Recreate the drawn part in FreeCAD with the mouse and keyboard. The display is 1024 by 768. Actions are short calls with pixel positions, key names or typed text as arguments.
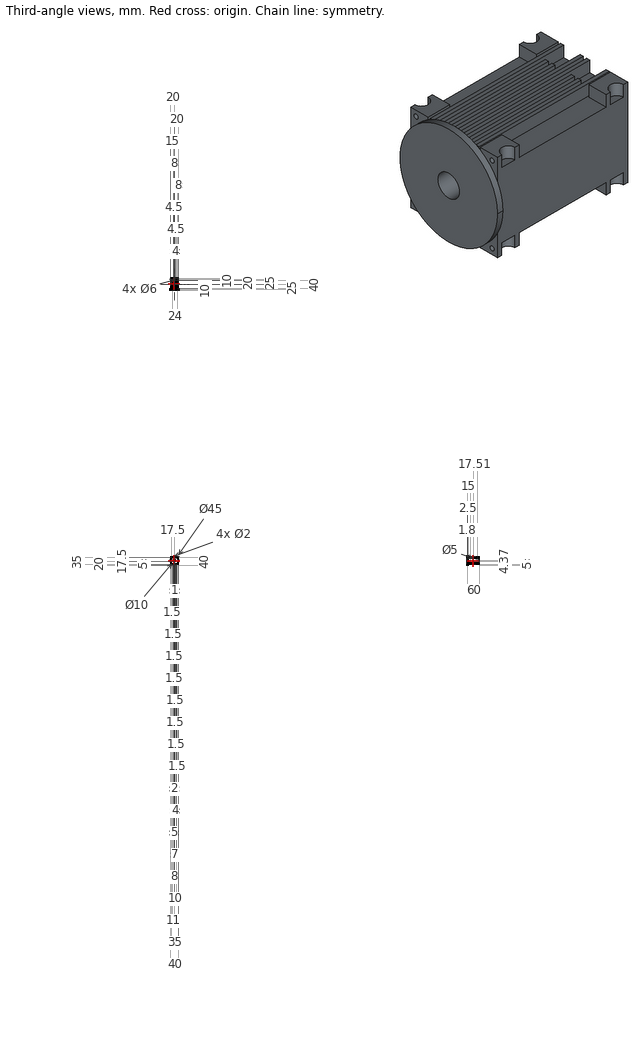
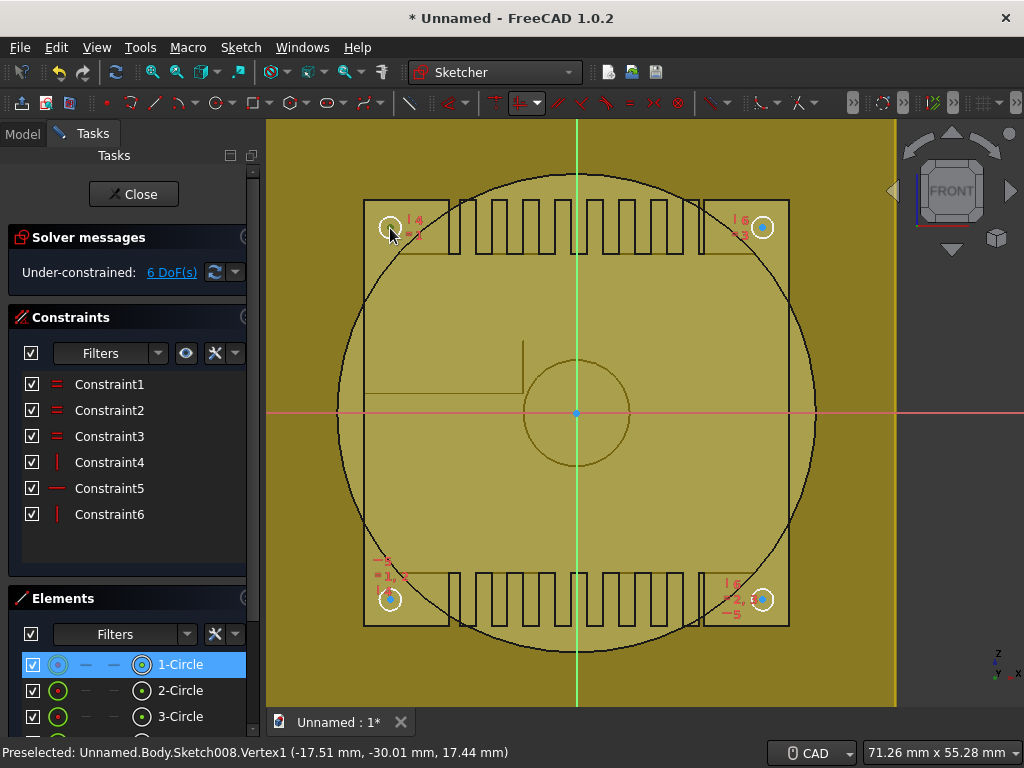
click(763, 228)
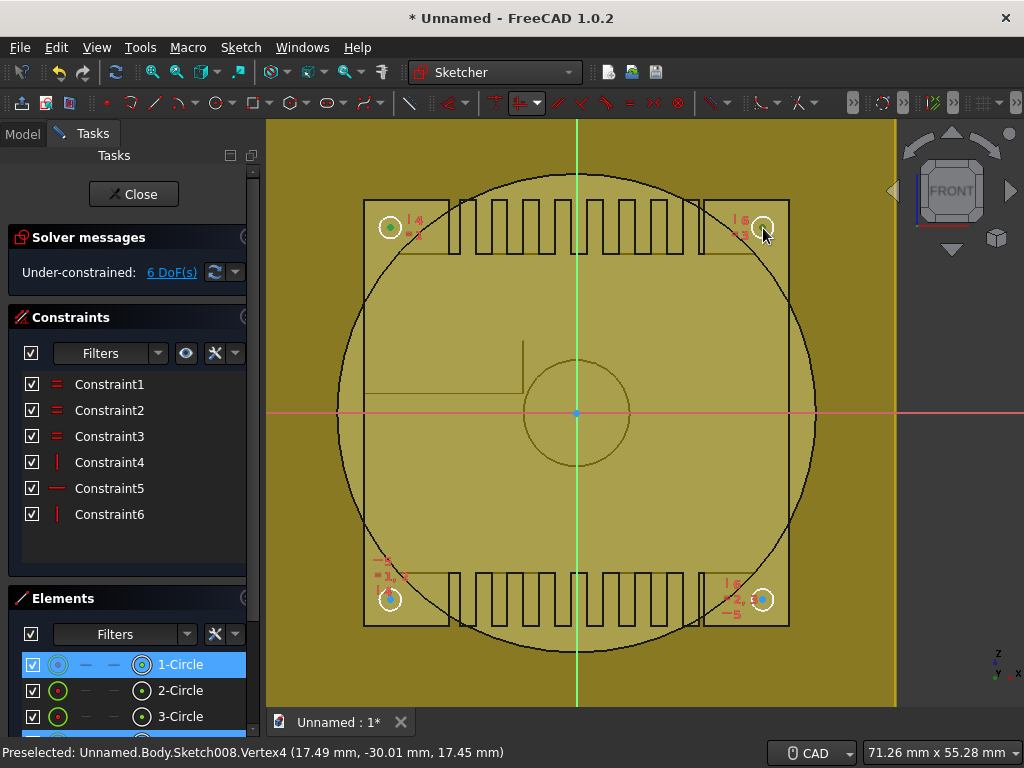
key(h)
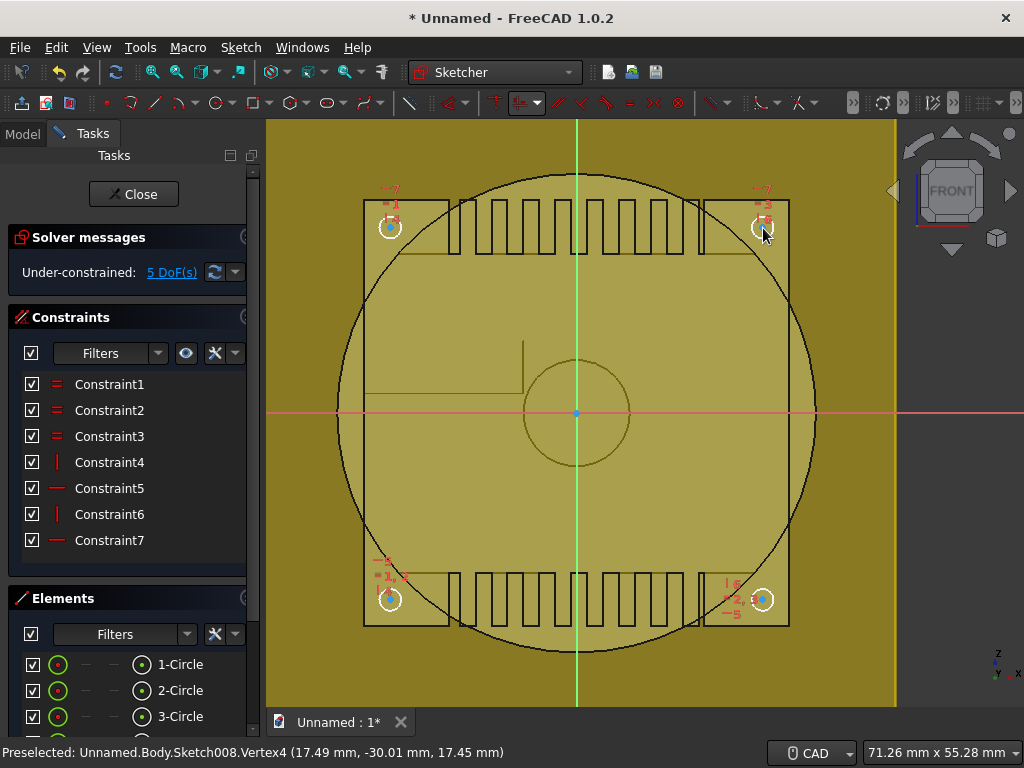
key(d)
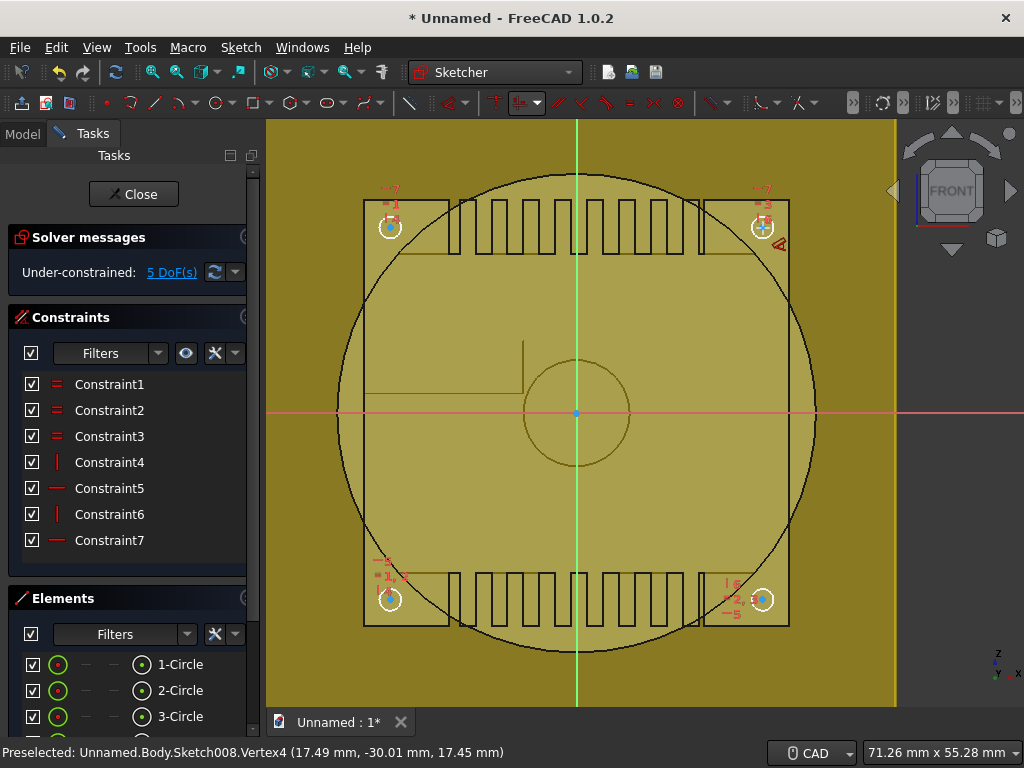
scroll(398, 220, up, 4)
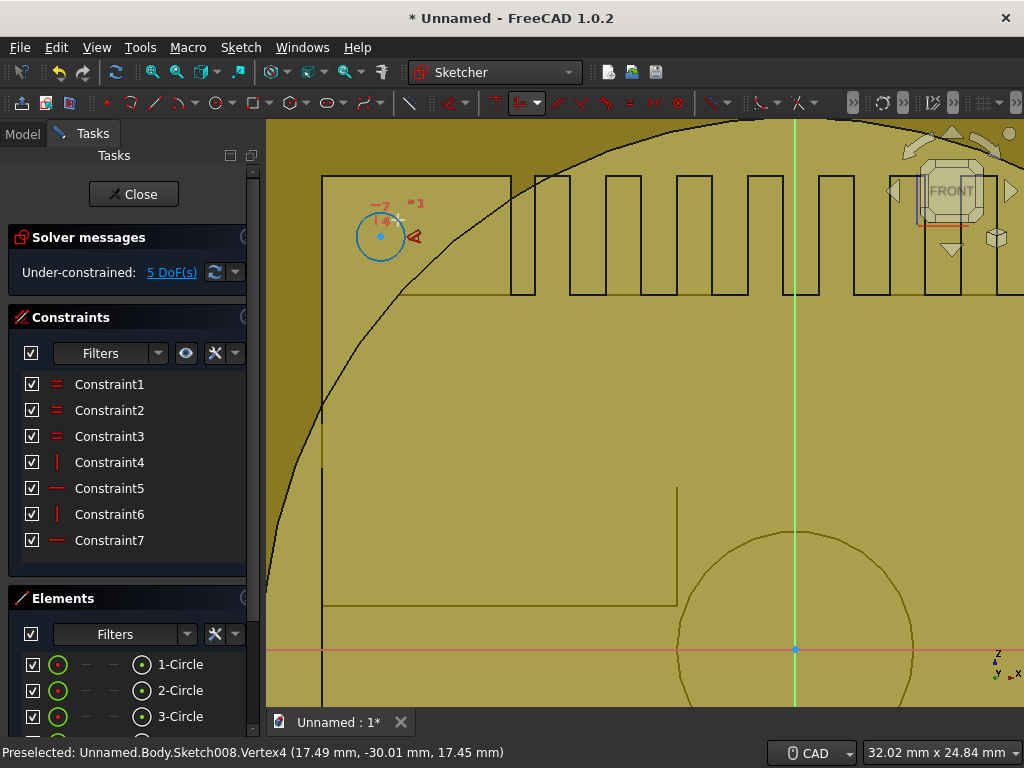
click(398, 220)
click(421, 198)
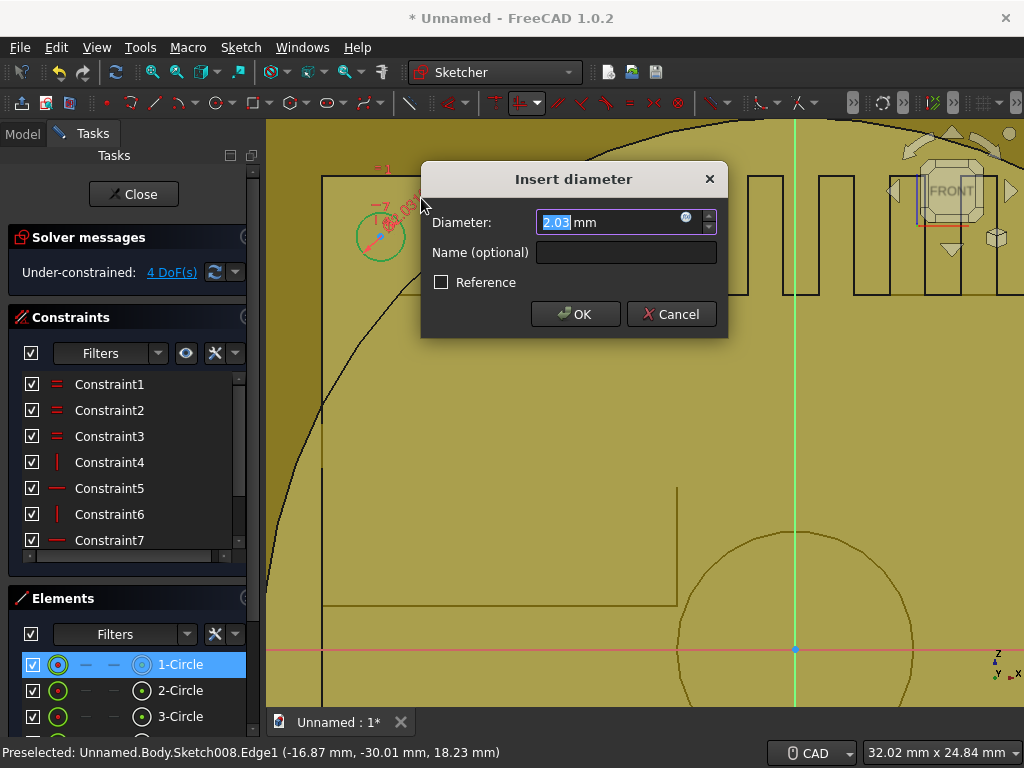
text(2)
key(Return)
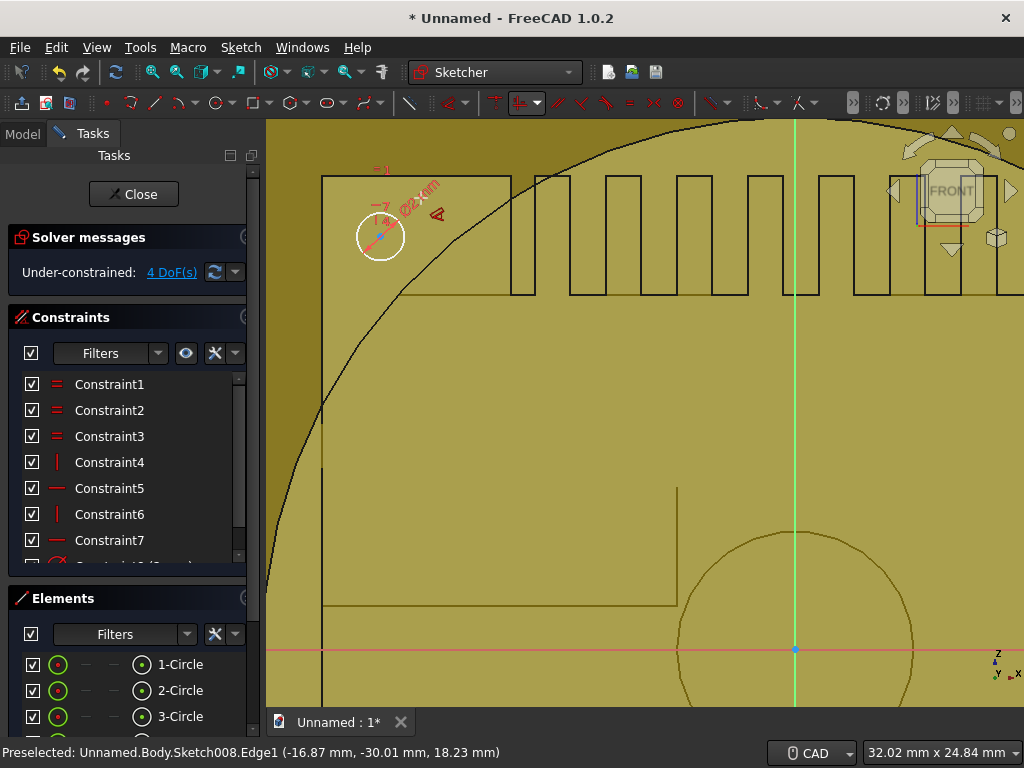
click(381, 237)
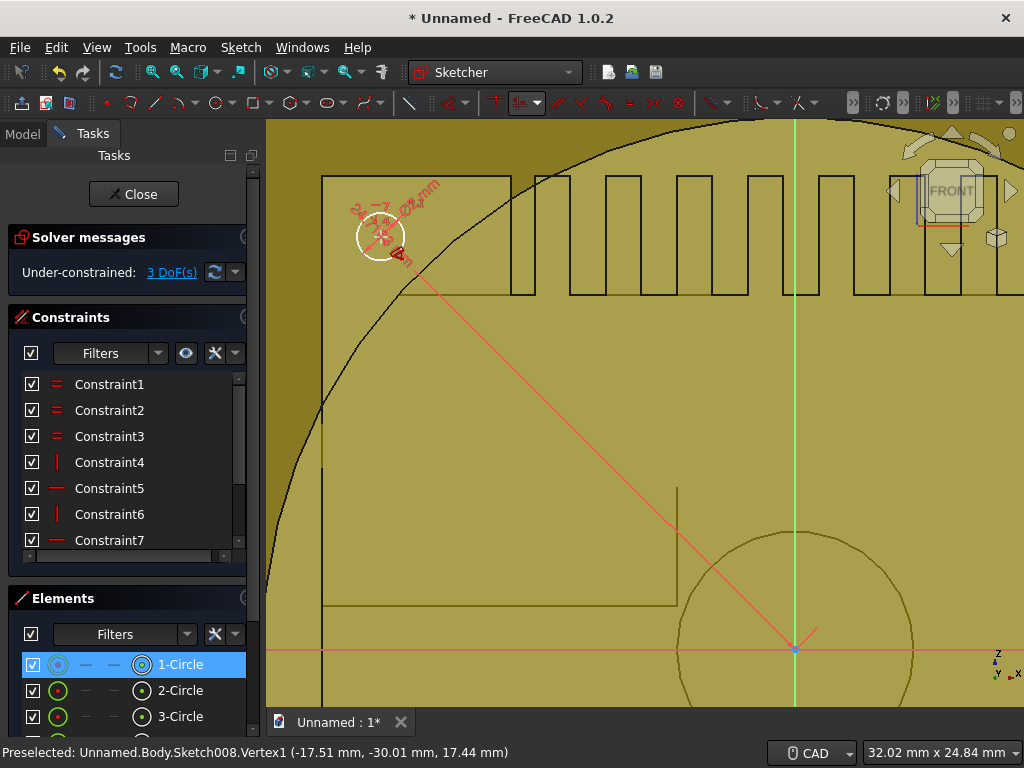
scroll(398, 220, down, 4)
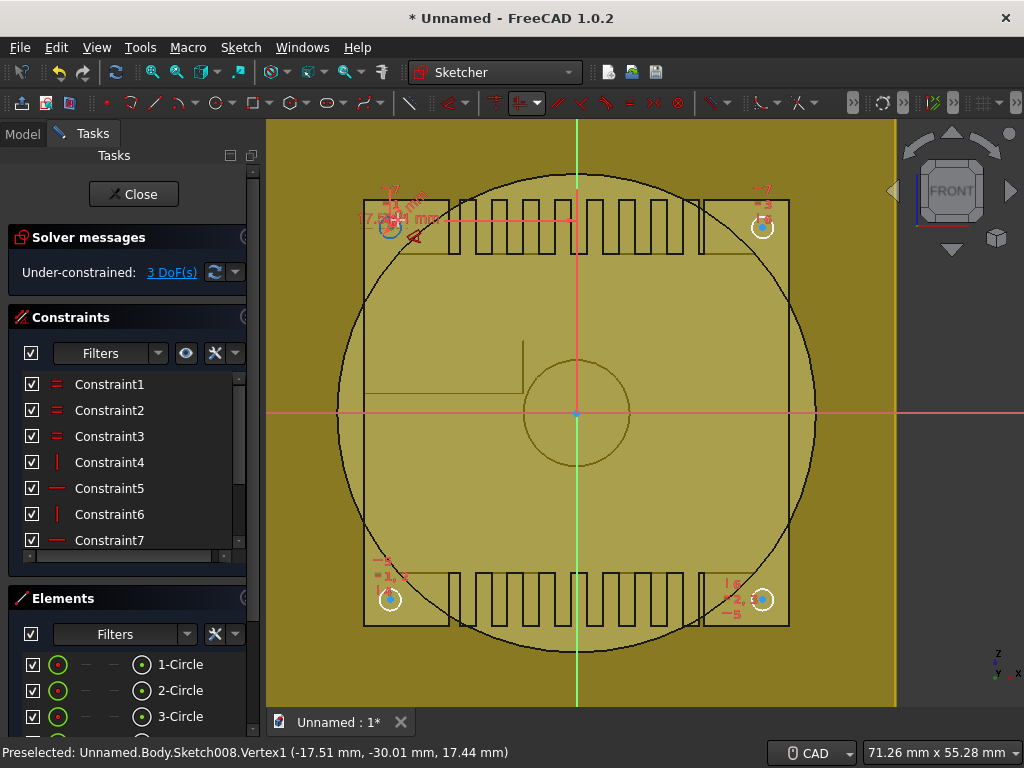
click(390, 600)
click(356, 328)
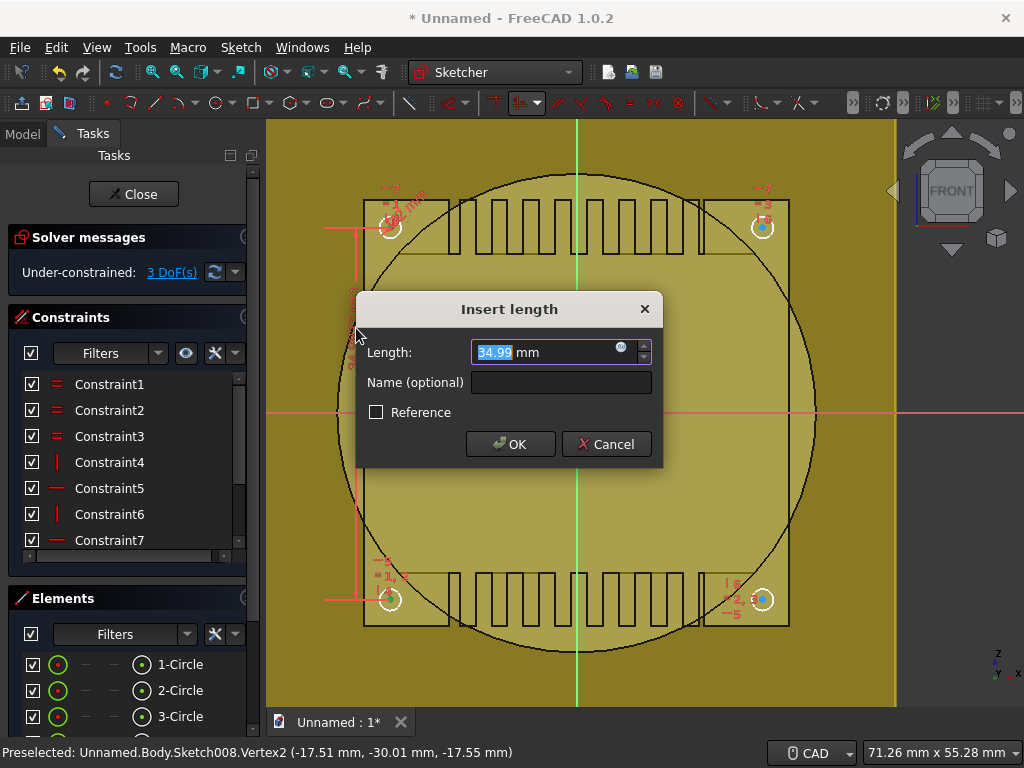
text(35)
key(Return)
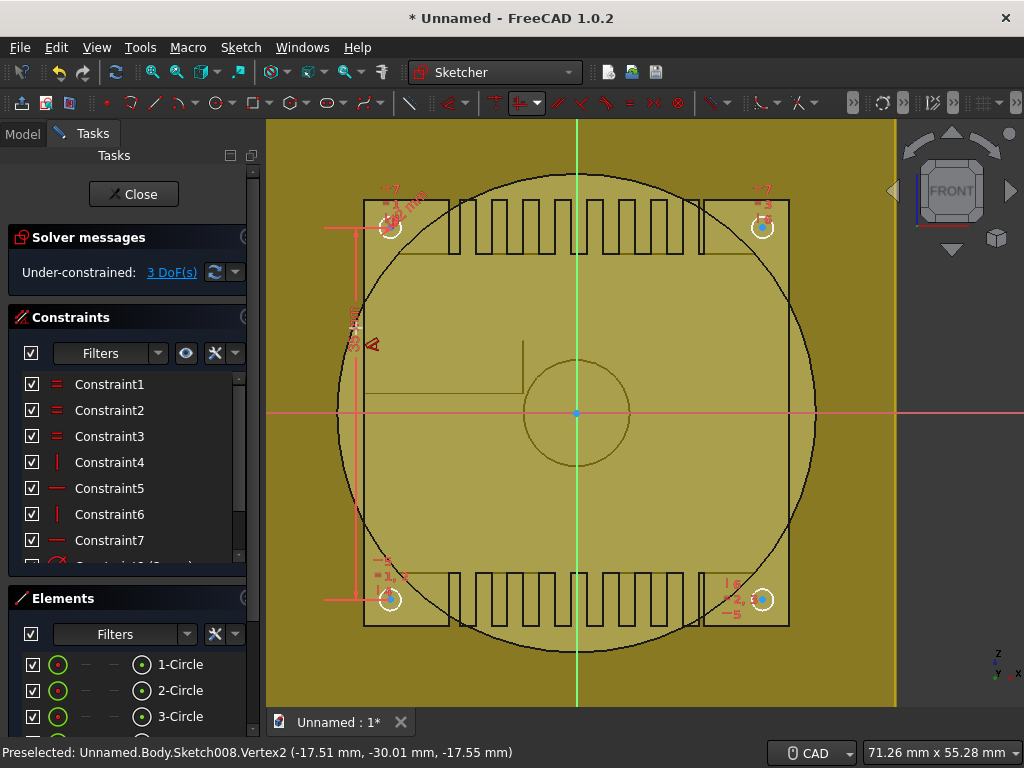
click(390, 600)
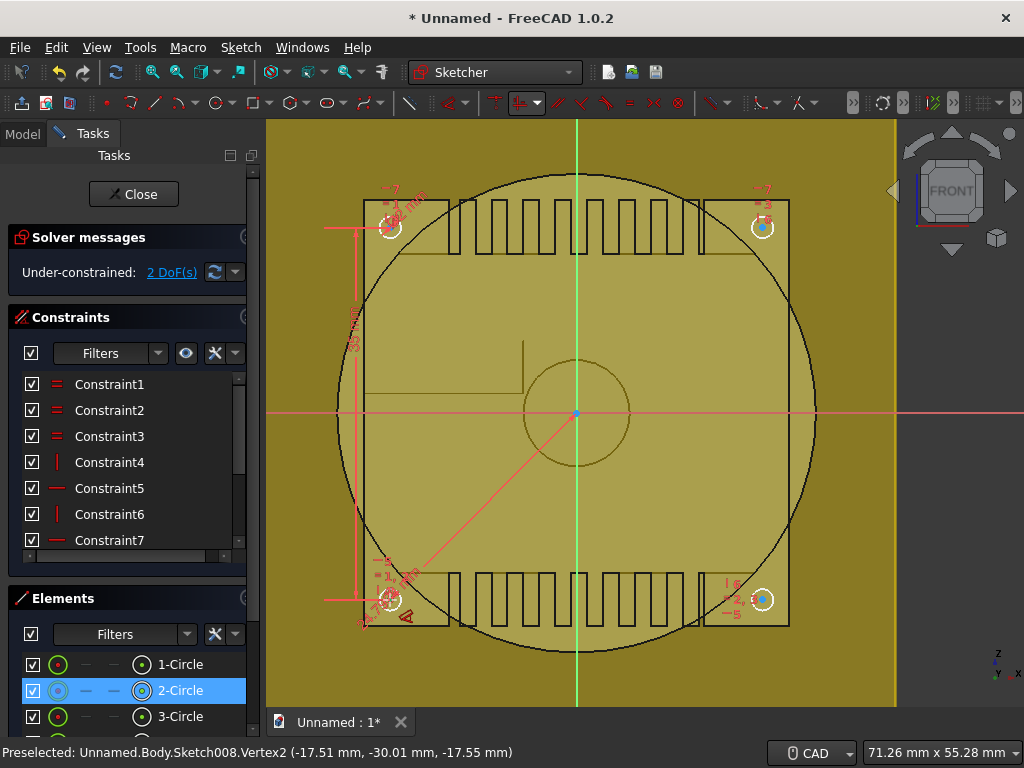
click(763, 600)
click(491, 634)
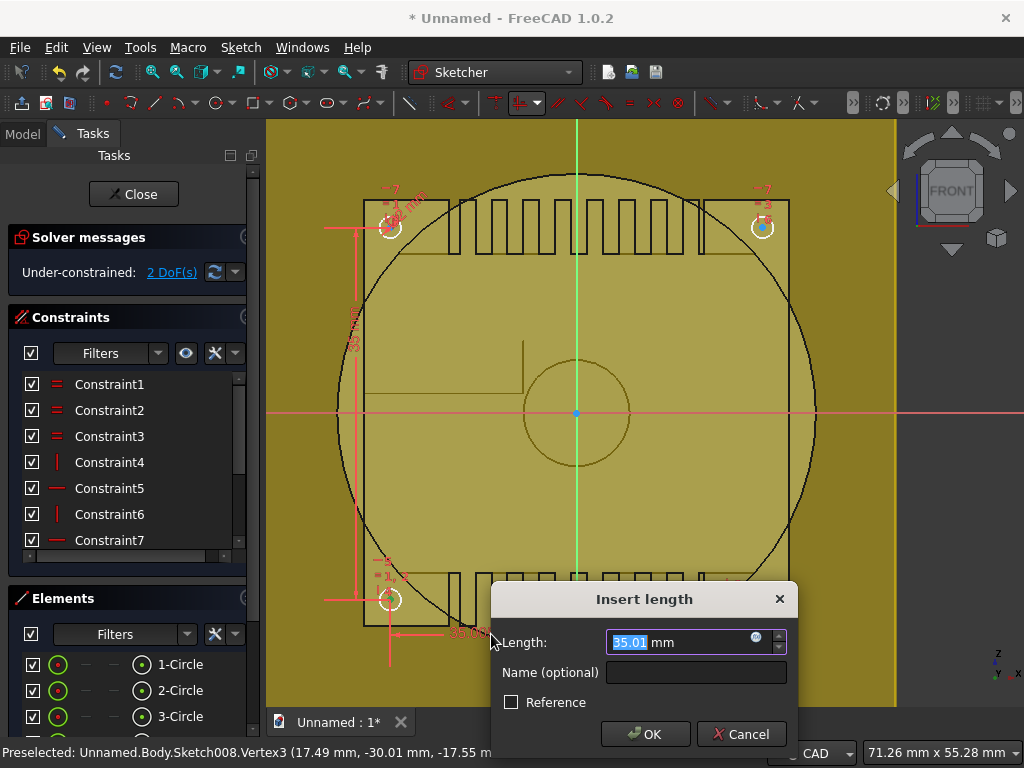
text(35)
key(Return)